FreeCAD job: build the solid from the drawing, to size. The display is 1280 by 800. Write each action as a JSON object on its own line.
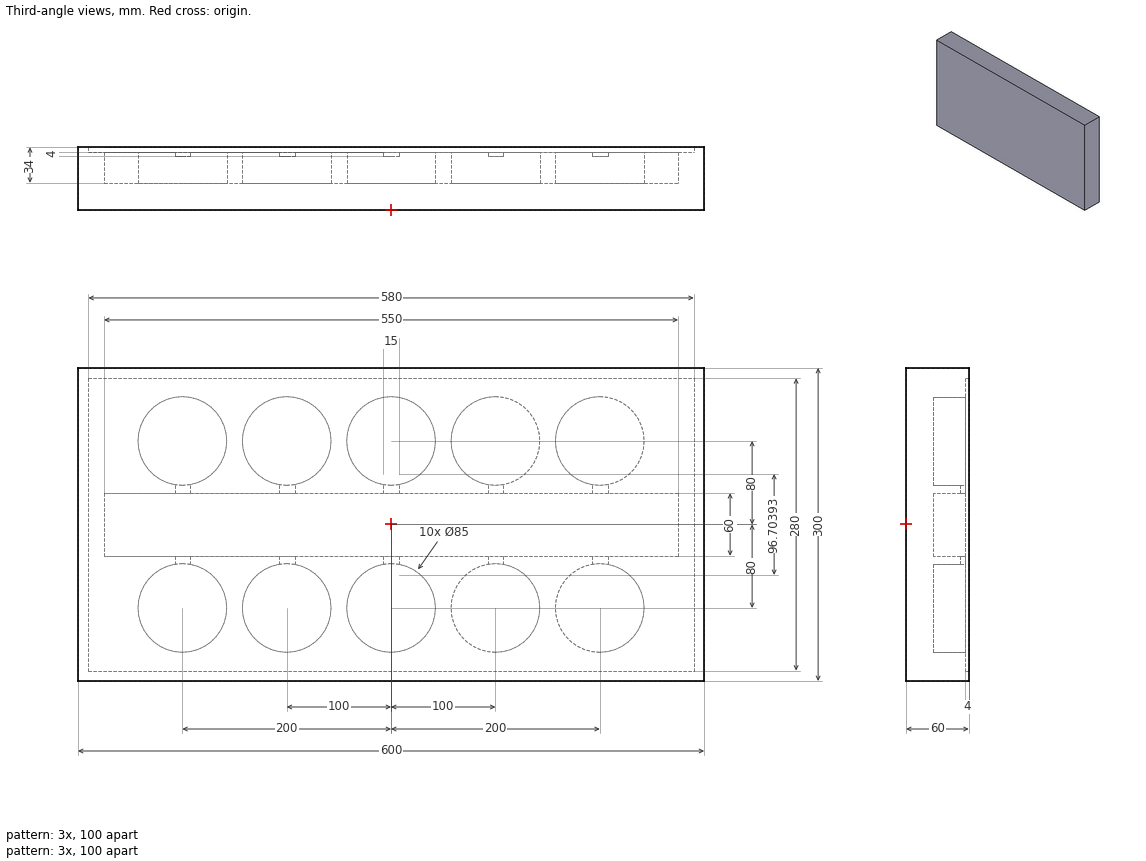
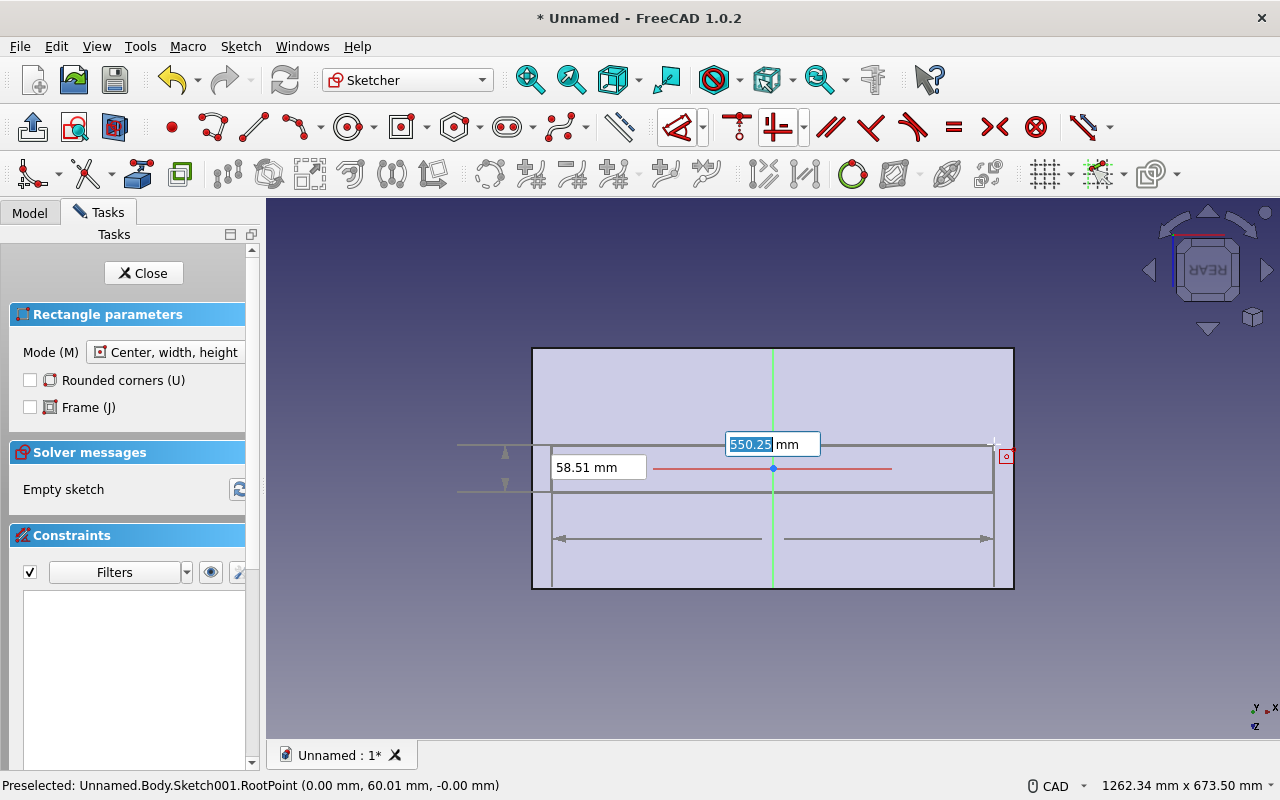
{"action": "type", "text": "550"}
{"action": "key", "text": "Tab"}
{"action": "type", "text": "60"}
{"action": "key", "text": "Return"}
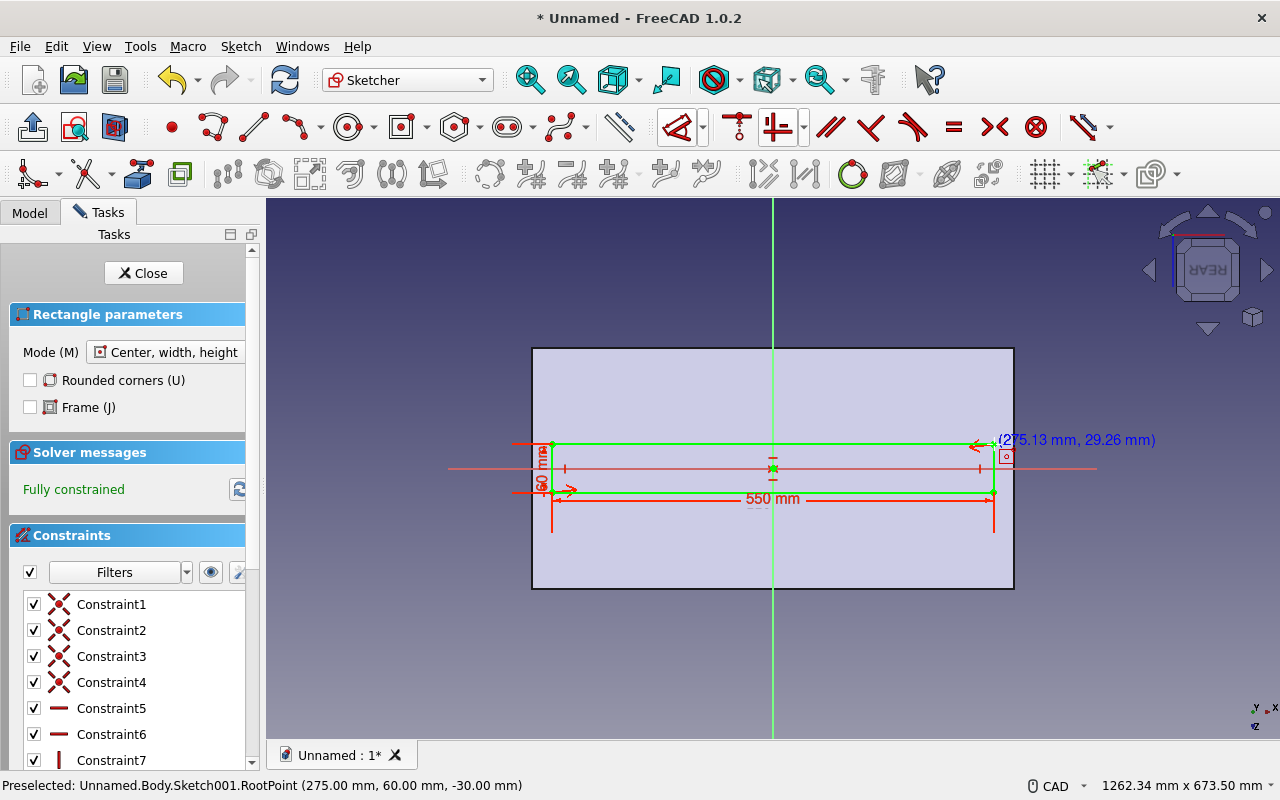
{"action": "left_click", "coordinate": [348, 128]}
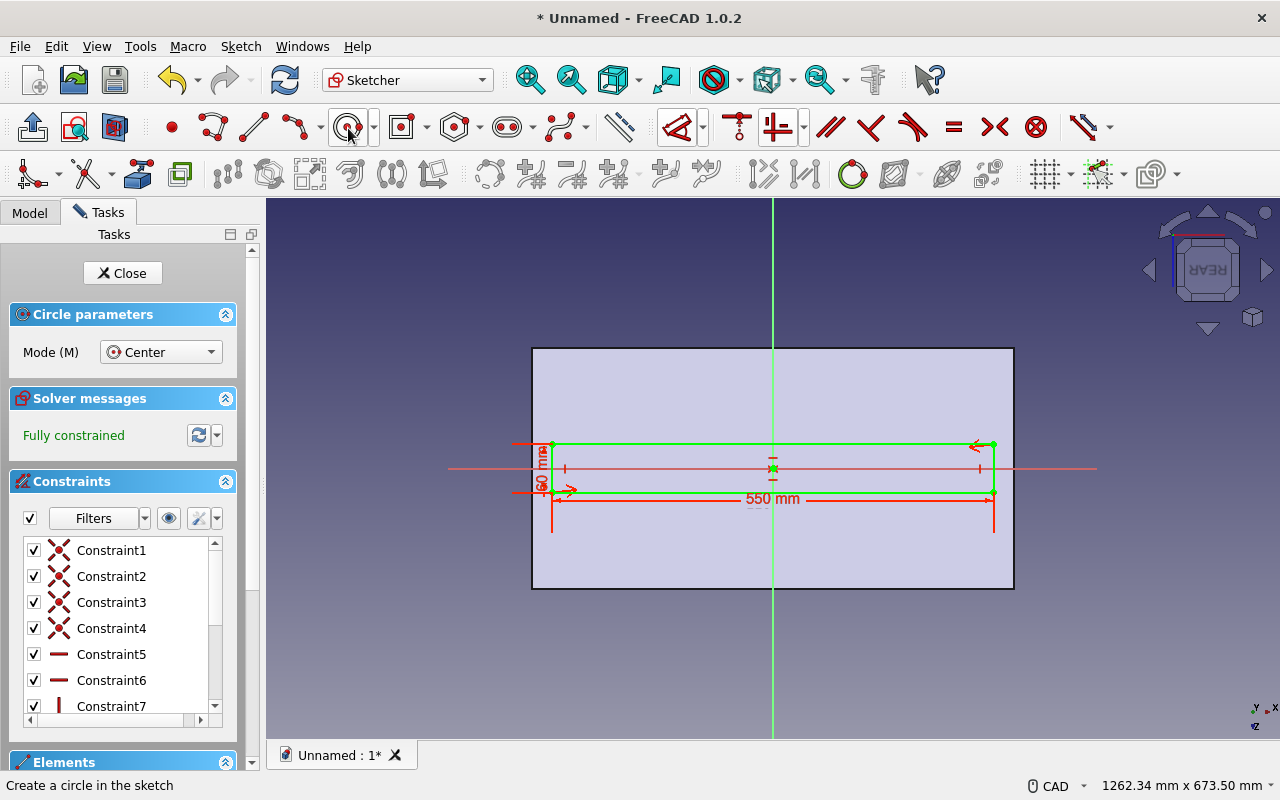
{"action": "left_click", "coordinate": [773, 404]}
{"action": "mouse_move", "coordinate": [797, 380]}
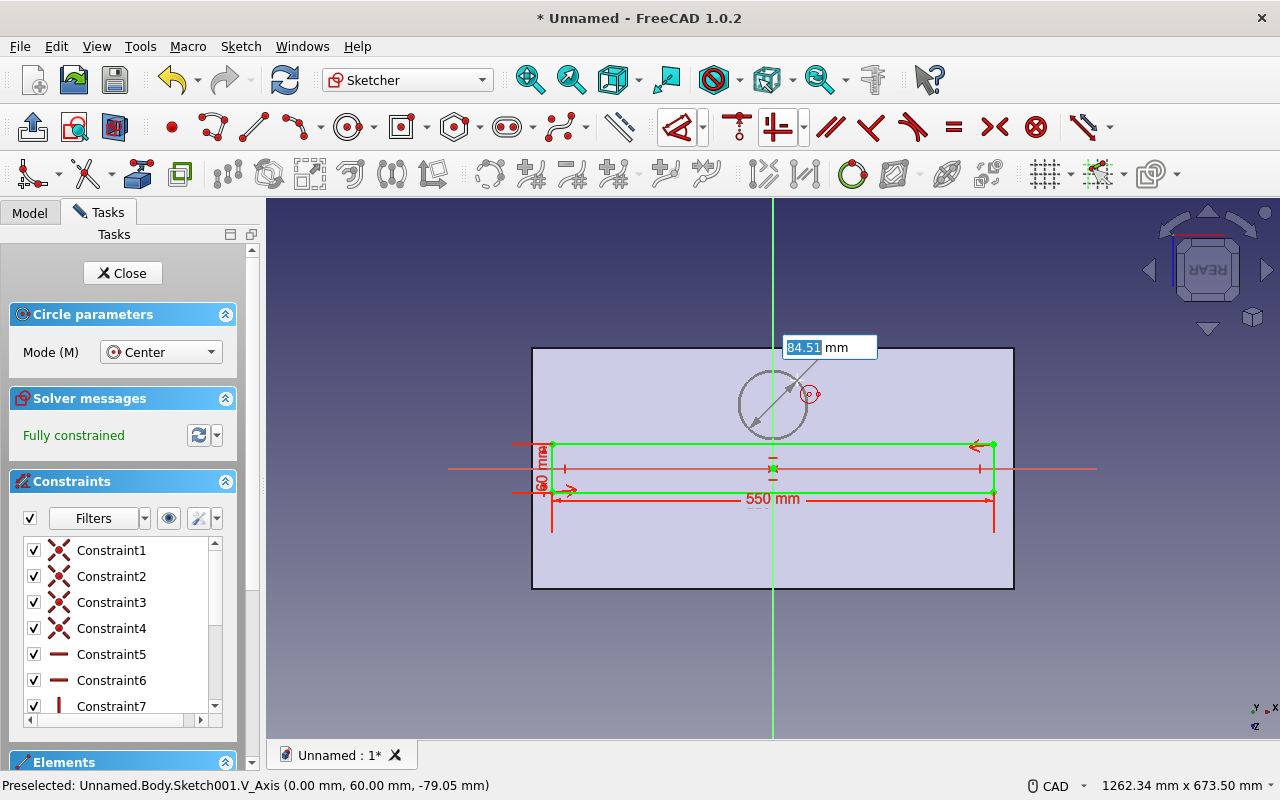
{"action": "type", "text": "85"}
{"action": "key", "text": "Return"}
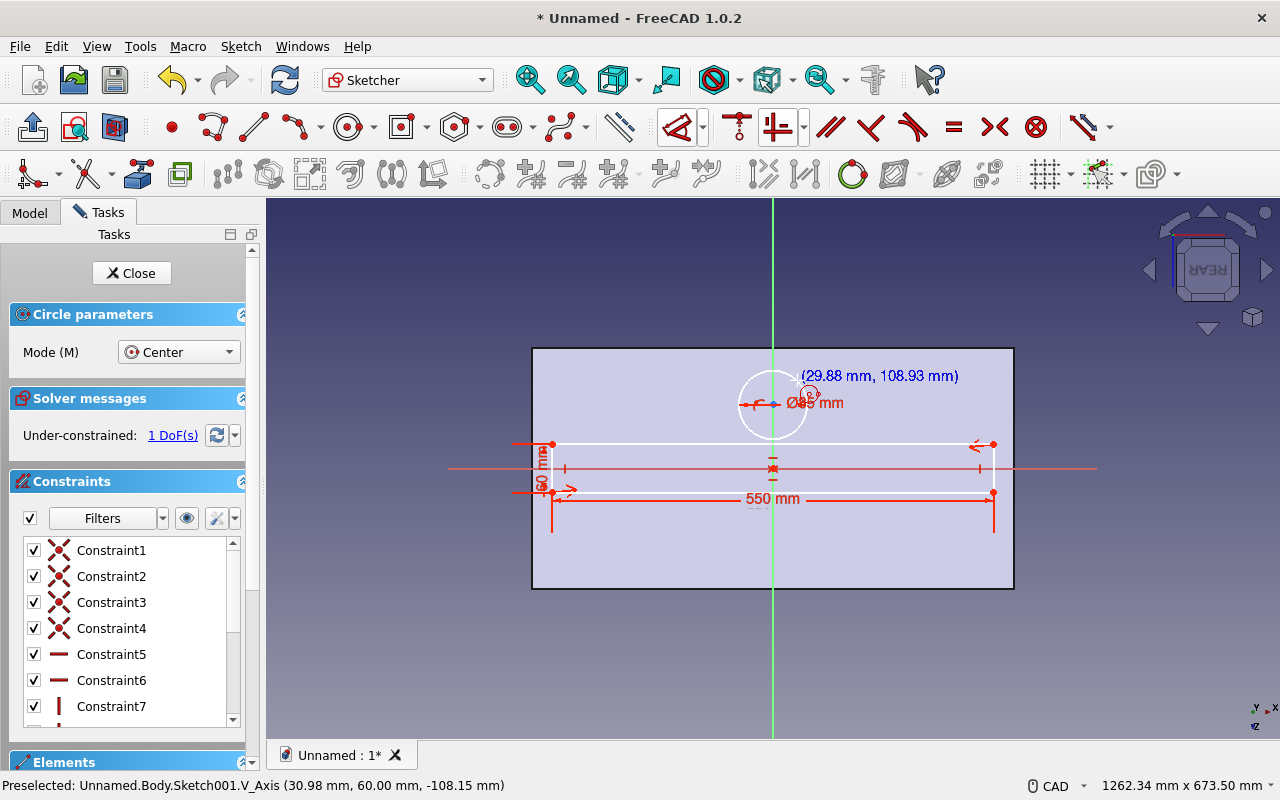
{"action": "left_click", "coordinate": [773, 533]}
{"action": "mouse_move", "coordinate": [797, 509]}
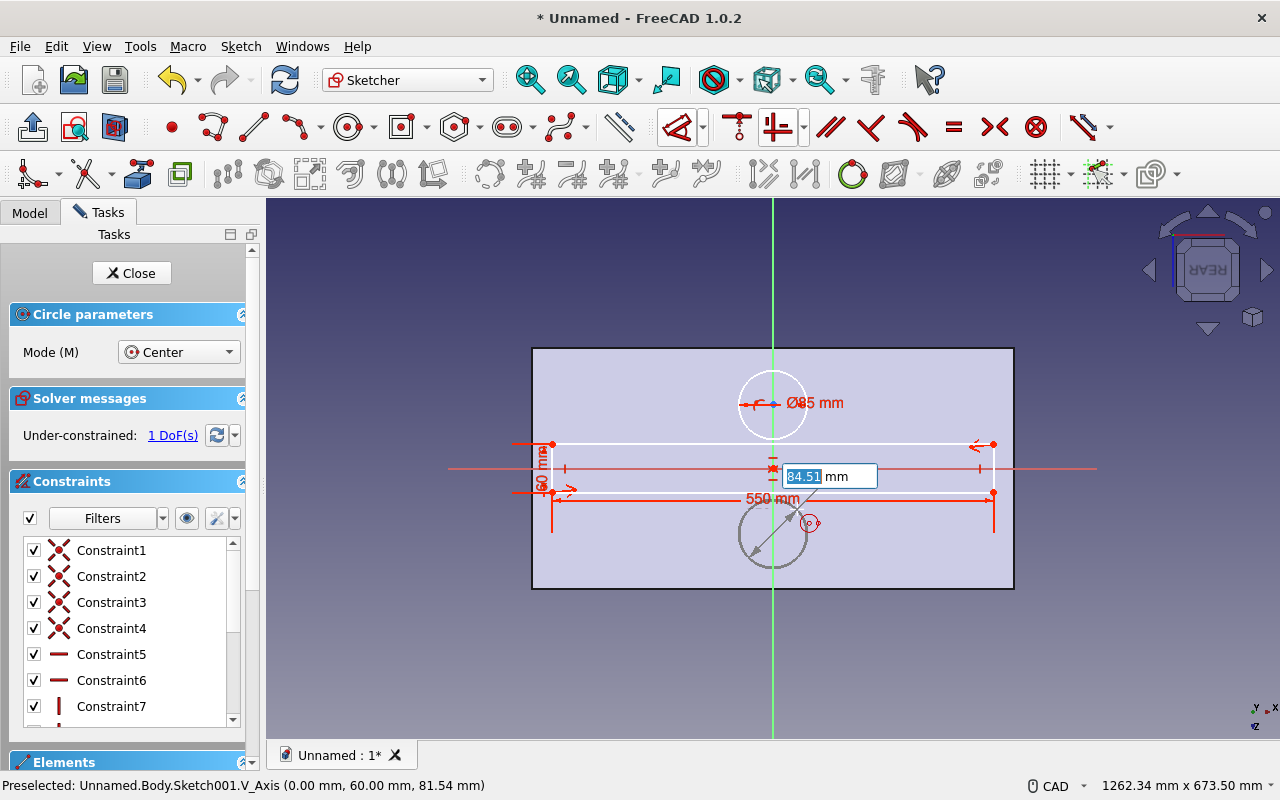
{"action": "type", "text": "85"}
{"action": "key", "text": "Return"}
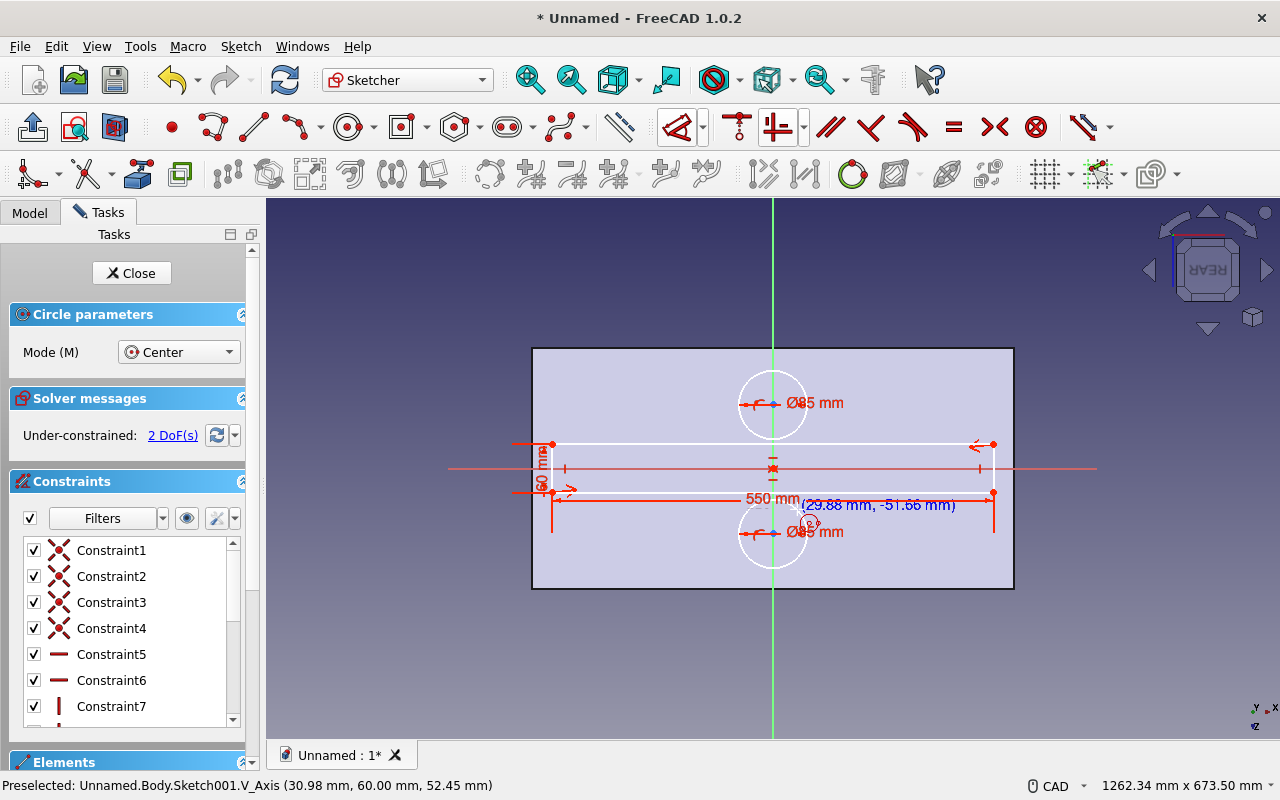
{"action": "left_click", "coordinate": [693, 404]}
{"action": "mouse_move", "coordinate": [717, 380]}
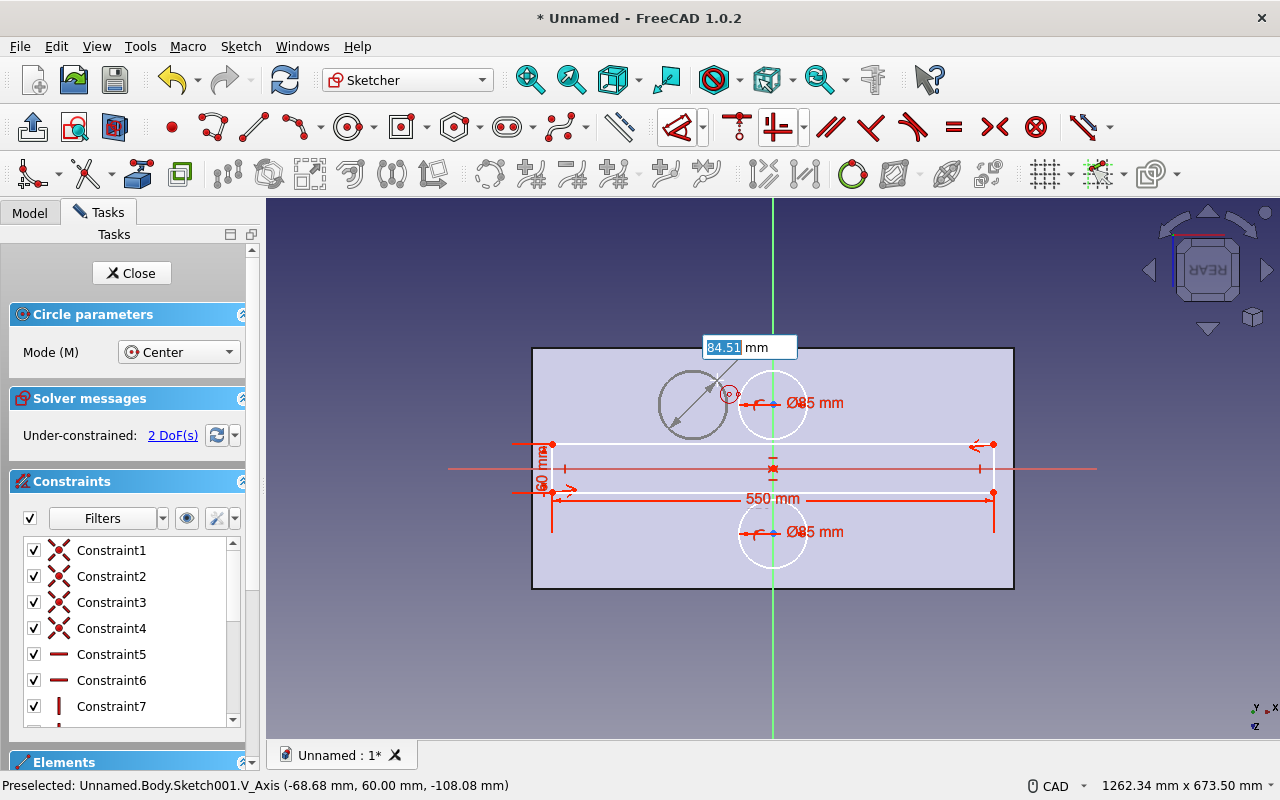
{"action": "type", "text": "85"}
{"action": "key", "text": "Return"}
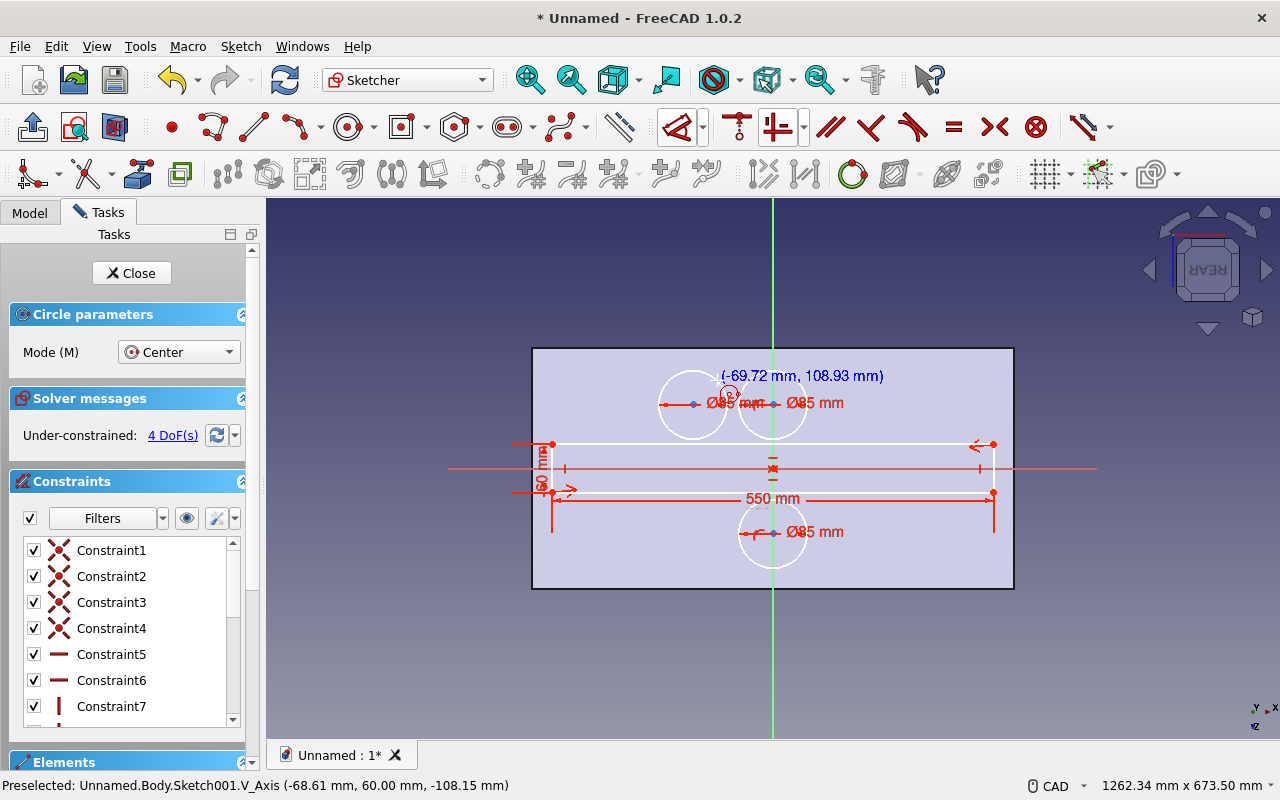
{"action": "left_click", "coordinate": [612, 404]}
{"action": "mouse_move", "coordinate": [636, 380]}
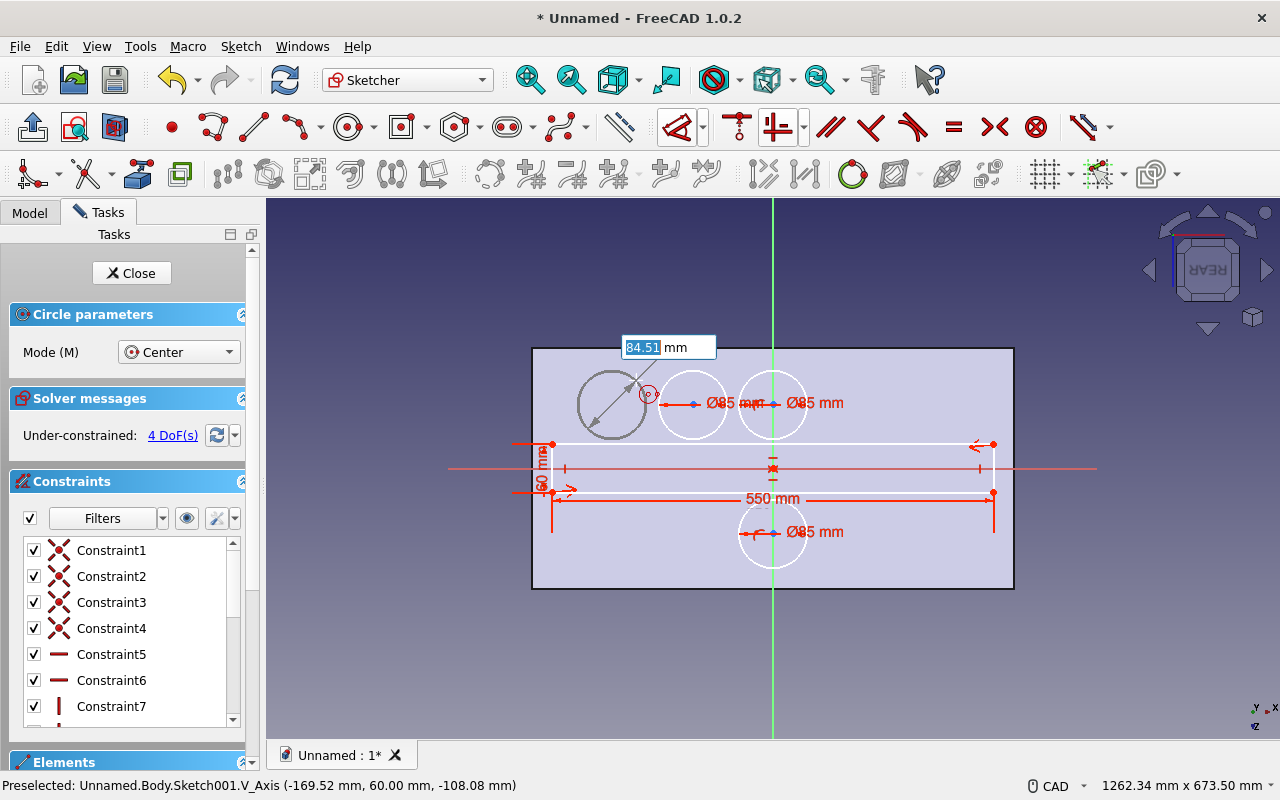
{"action": "type", "text": "85"}
{"action": "key", "text": "Return"}